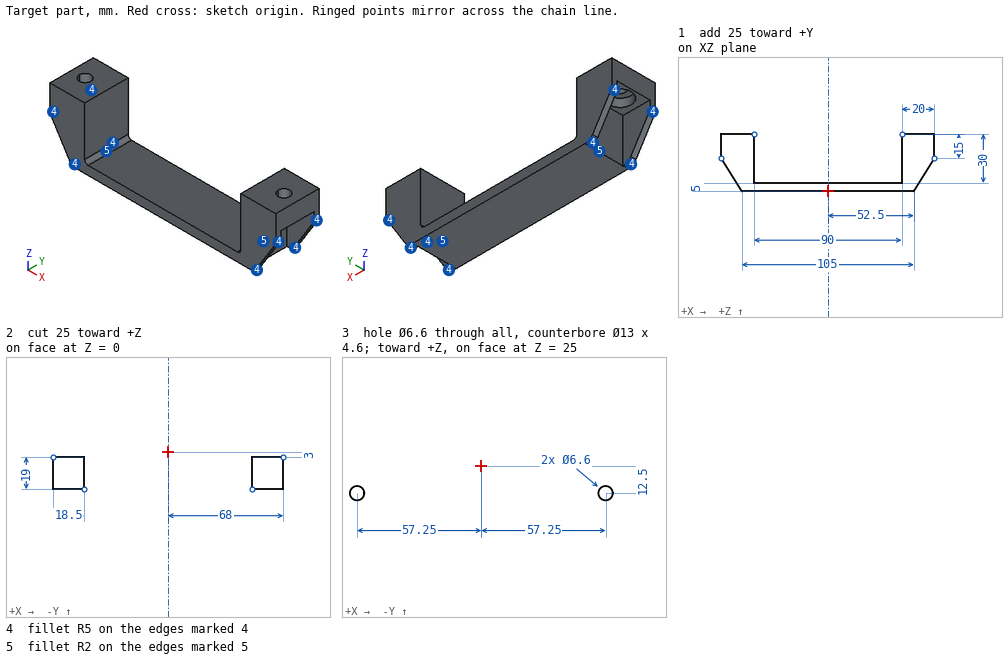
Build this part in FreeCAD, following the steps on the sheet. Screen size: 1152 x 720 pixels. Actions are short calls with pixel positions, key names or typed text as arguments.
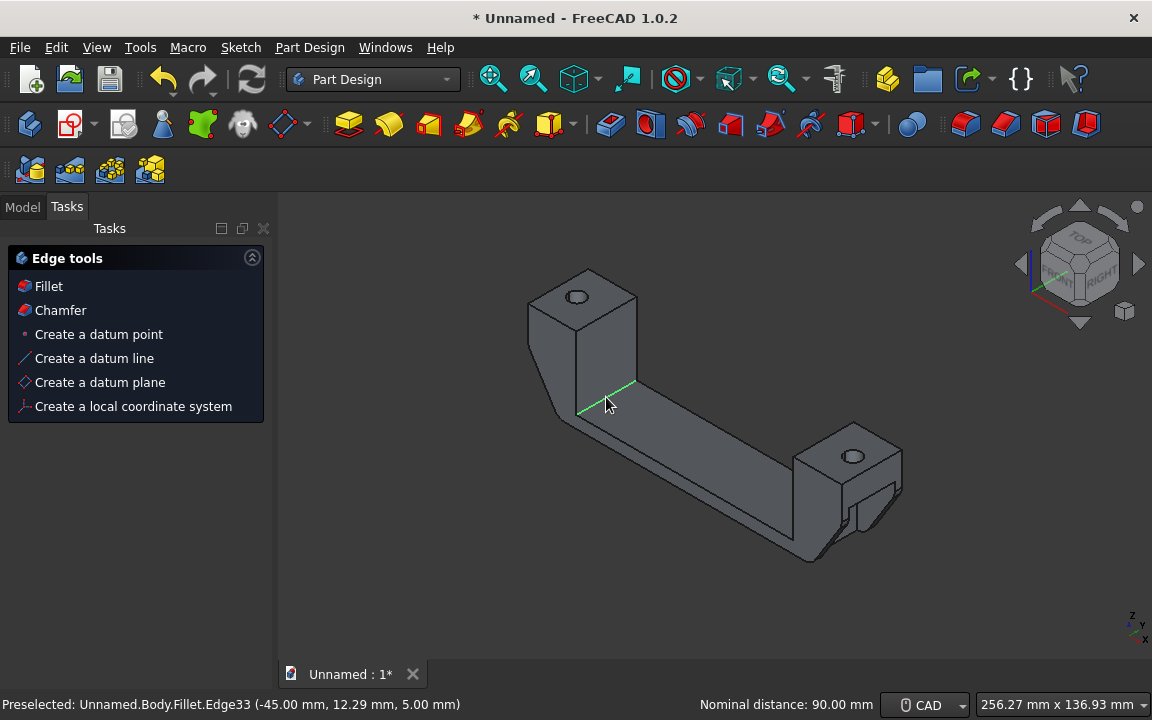
click(966, 124)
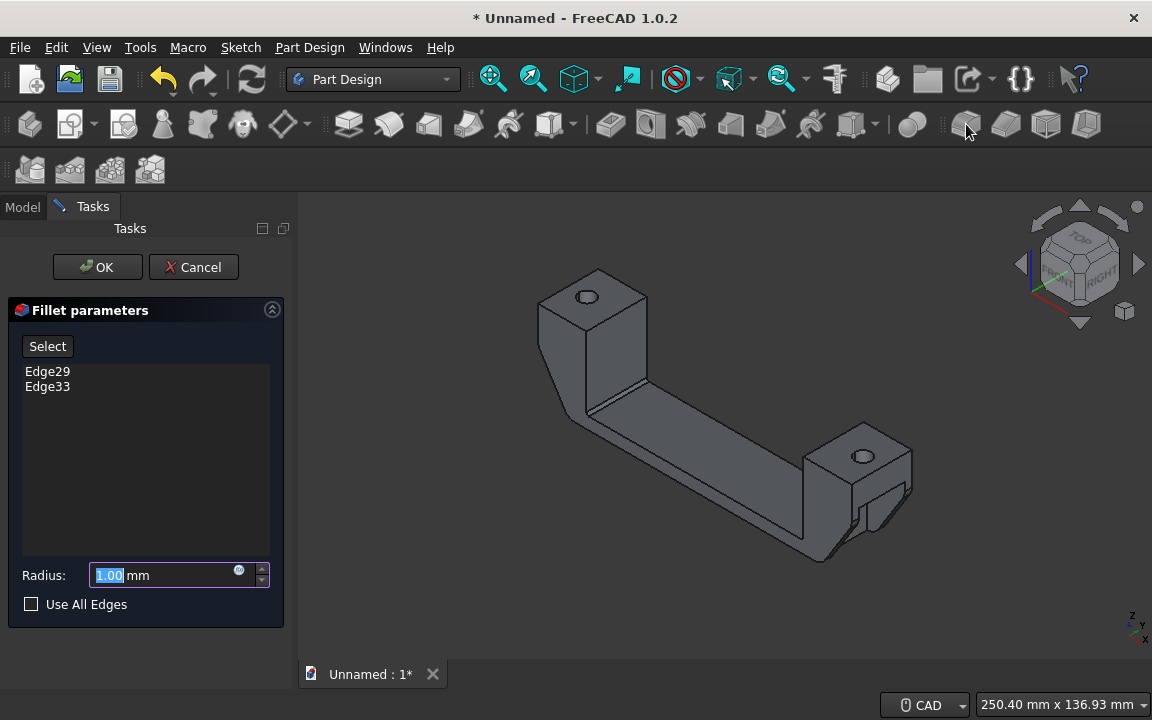
text(2)
key(Tab)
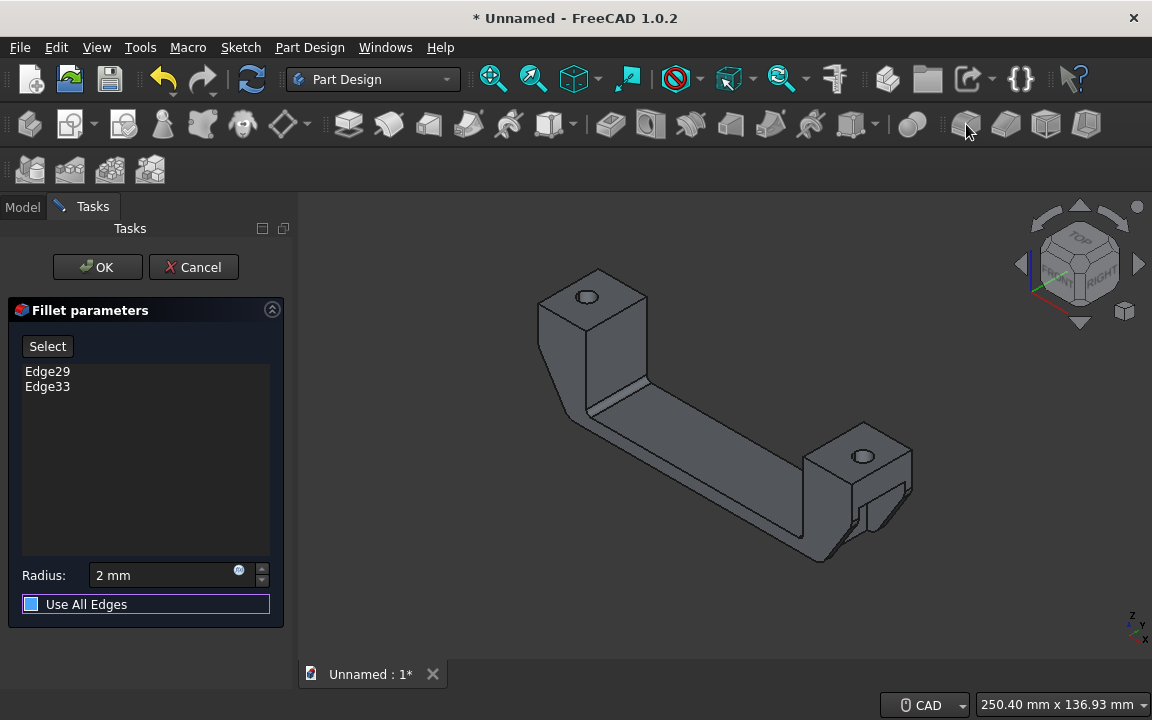
click(98, 267)